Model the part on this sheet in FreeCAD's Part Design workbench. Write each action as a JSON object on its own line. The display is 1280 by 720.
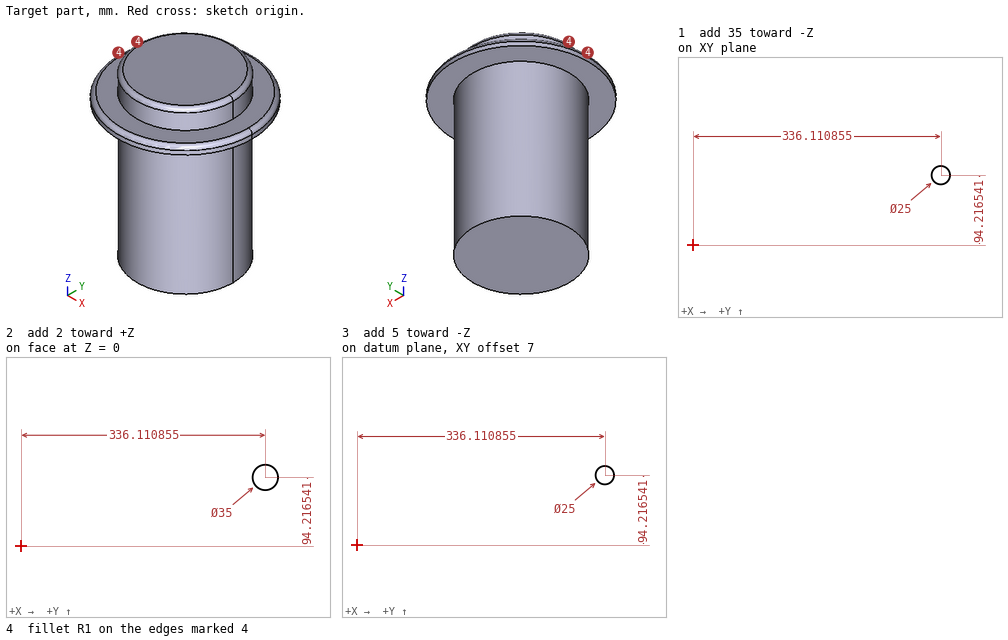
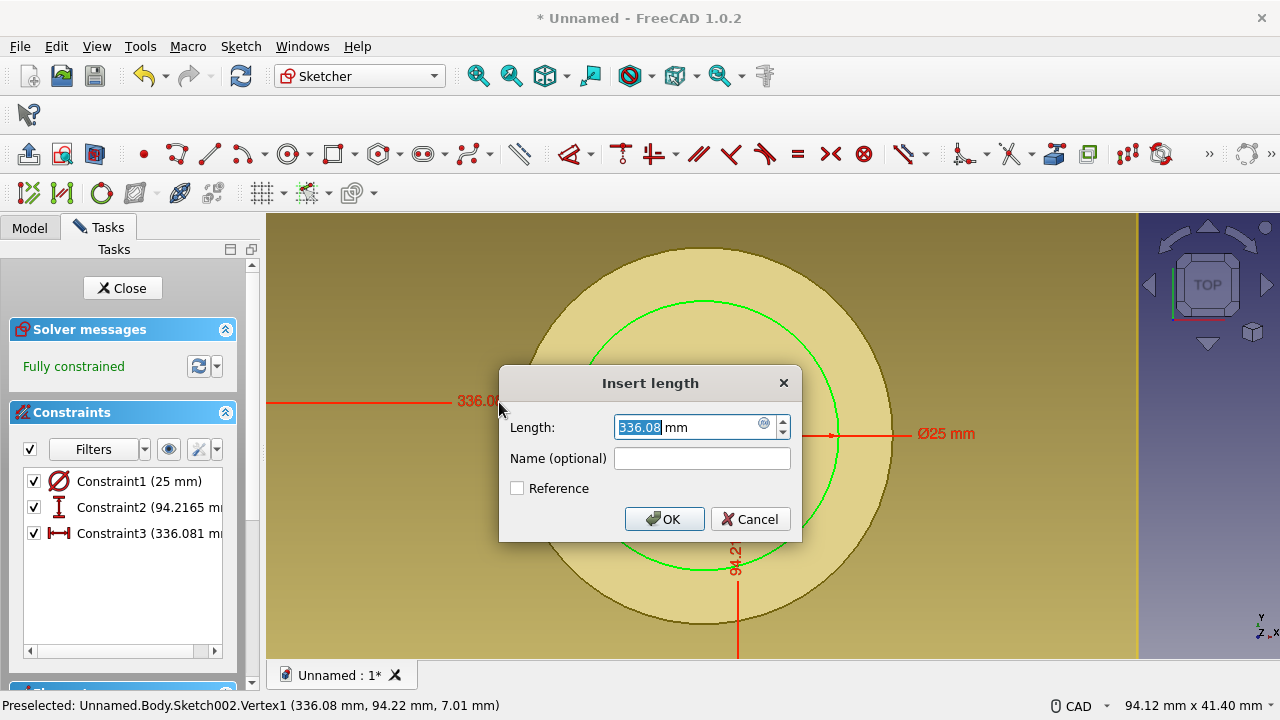
{"action": "type", "text": "336.110855"}
{"action": "key", "text": "Return"}
{"action": "key", "text": "Escape"}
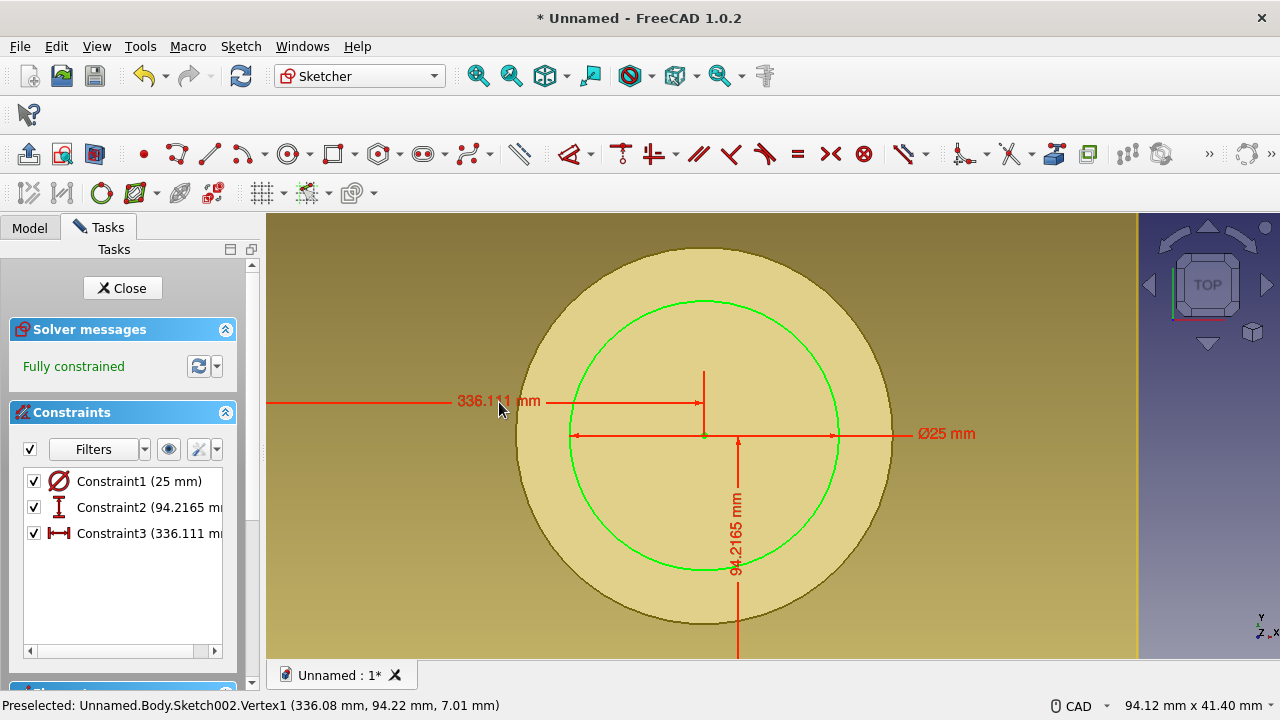
{"action": "left_click", "coordinate": [123, 288]}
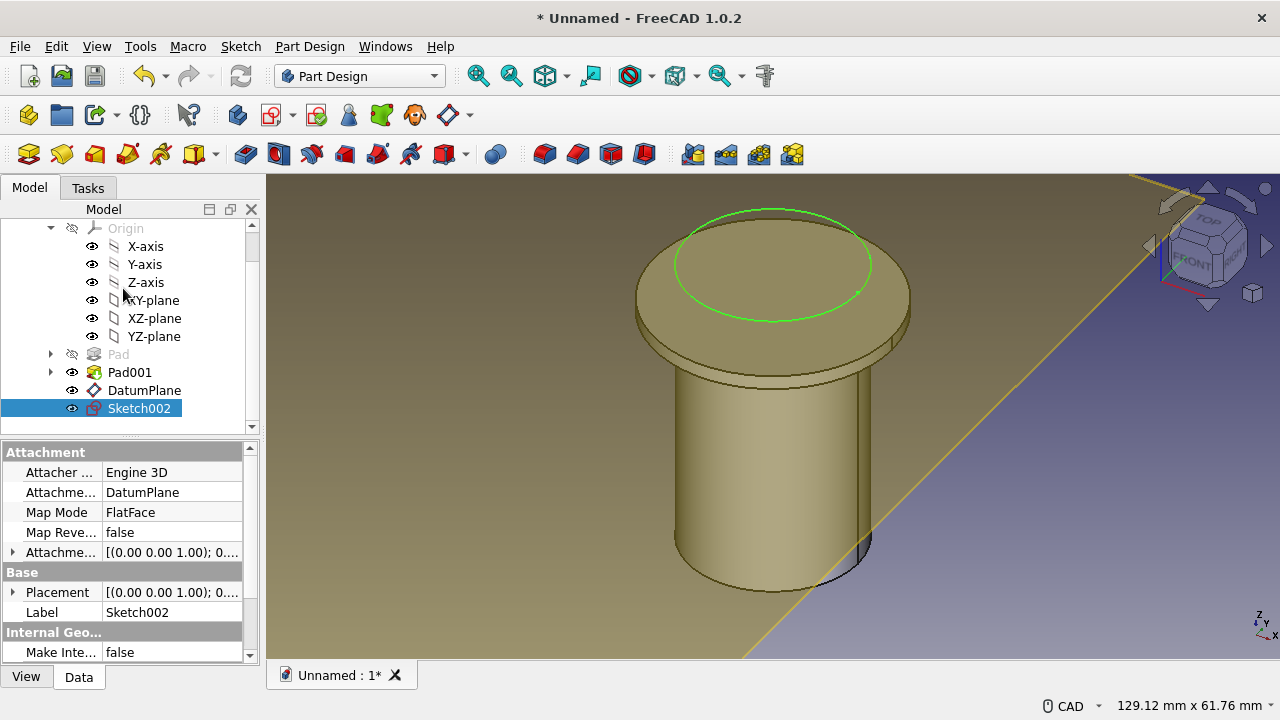
{"action": "left_click", "coordinate": [29, 154]}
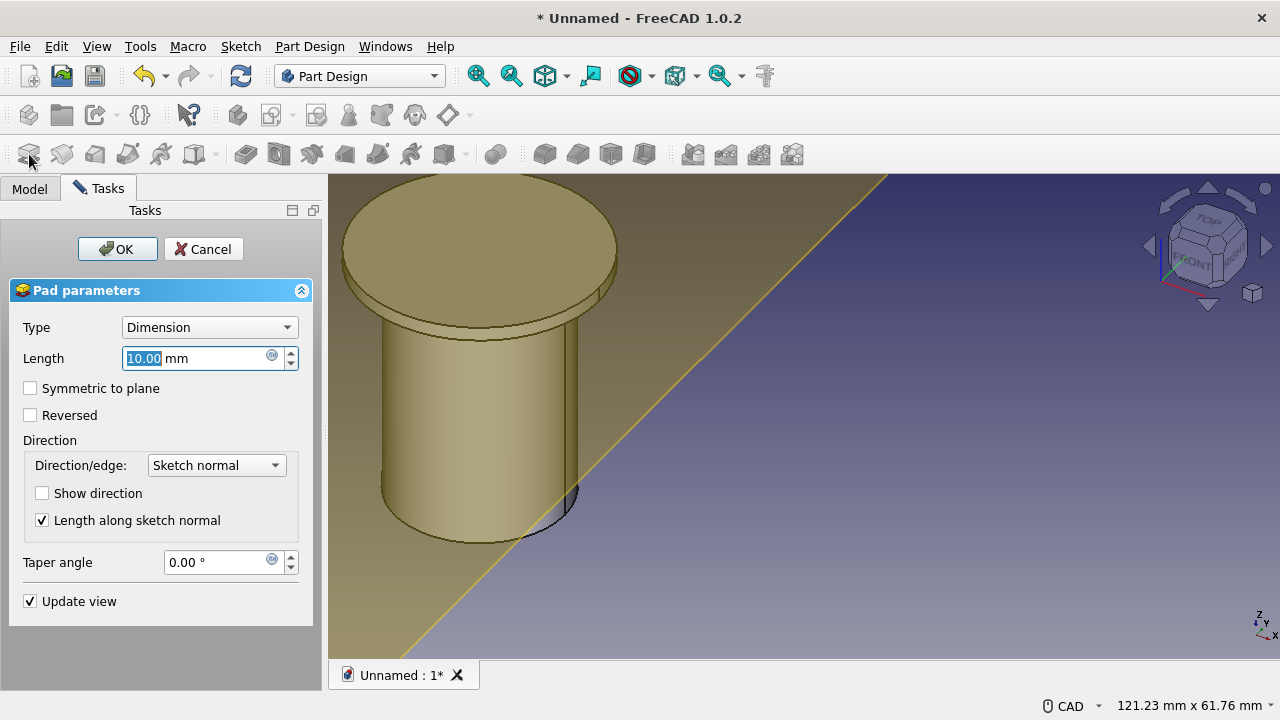
{"action": "type", "text": "5"}
{"action": "key", "text": "Tab"}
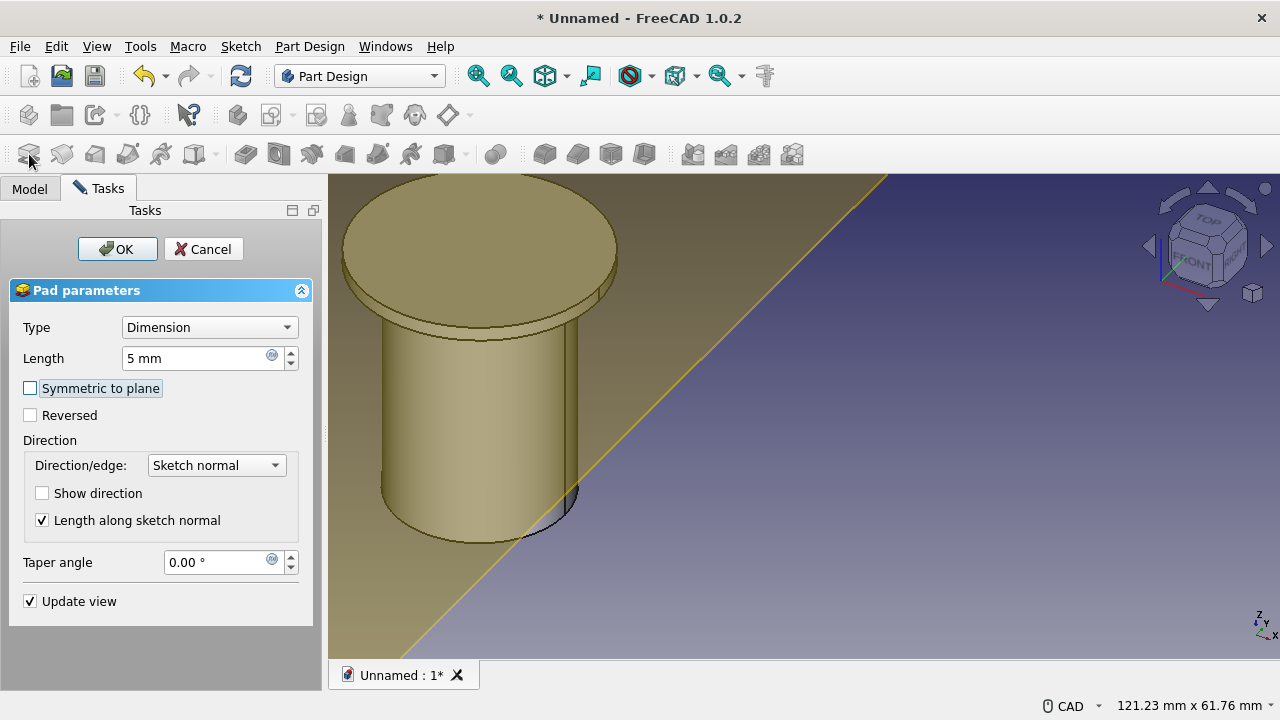
{"action": "left_click", "coordinate": [31, 415]}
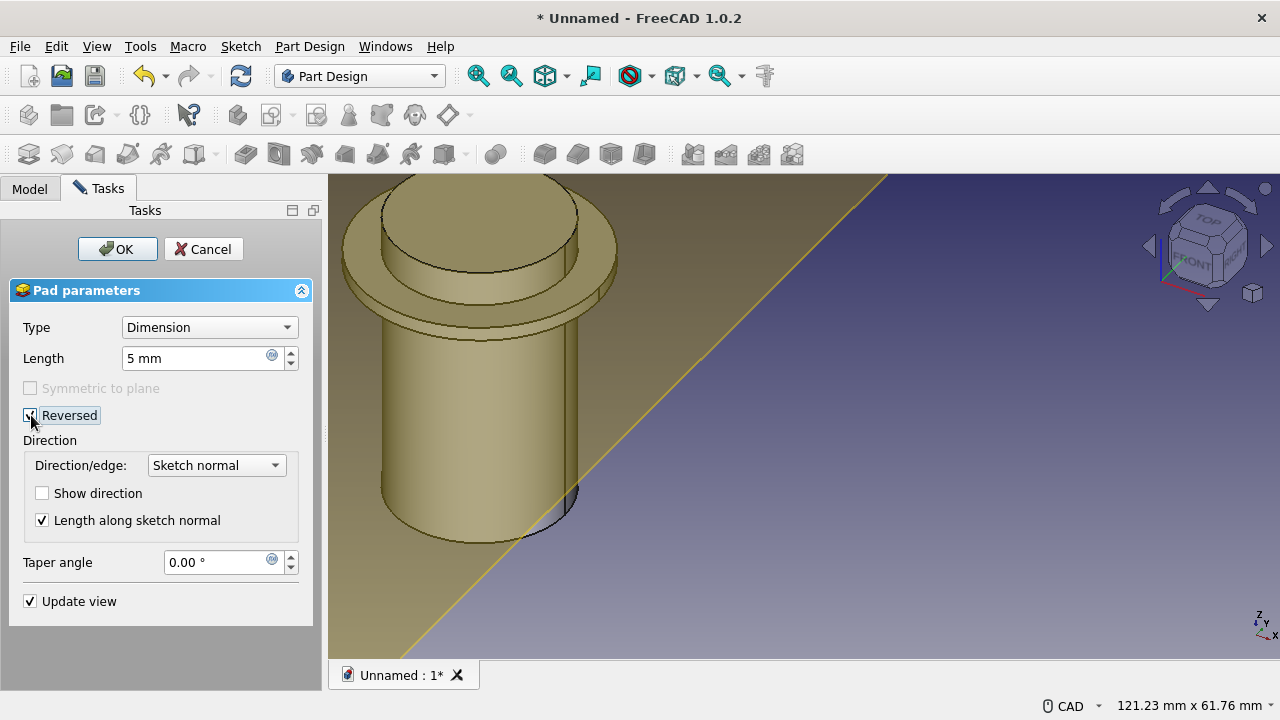
{"action": "left_click", "coordinate": [118, 249]}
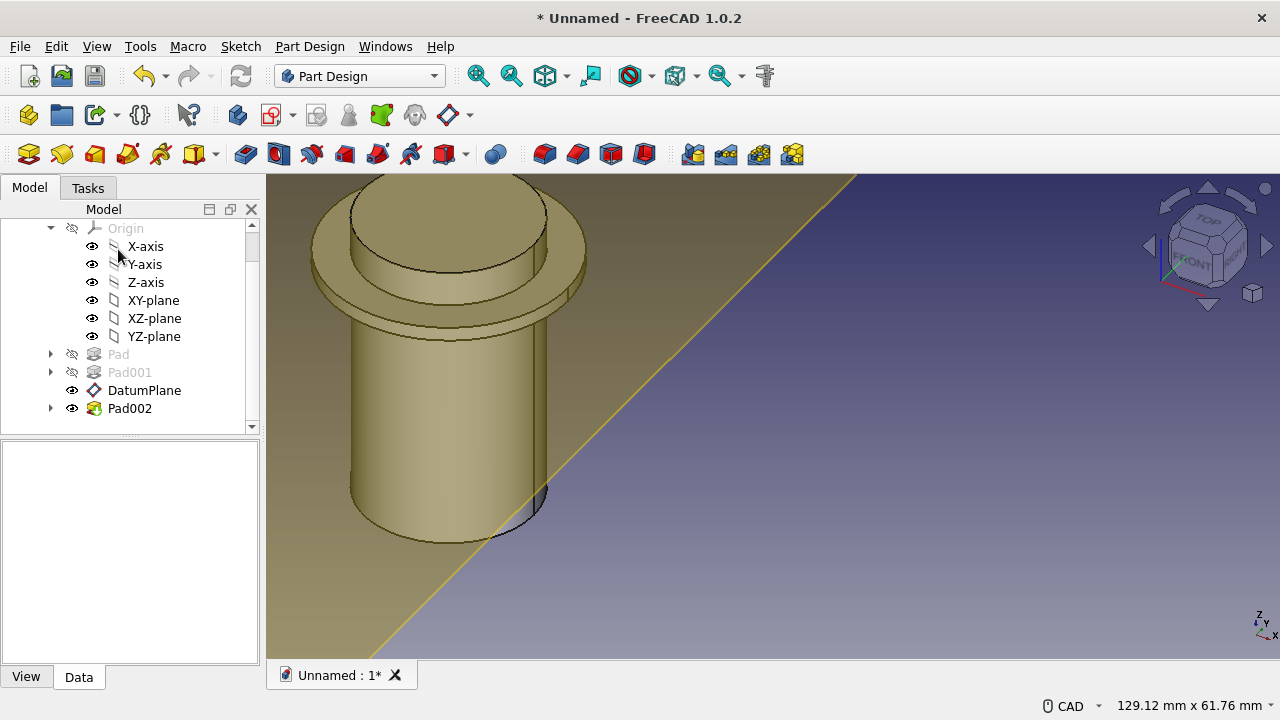
{"action": "left_click", "coordinate": [117, 390]}
{"action": "key", "text": "space"}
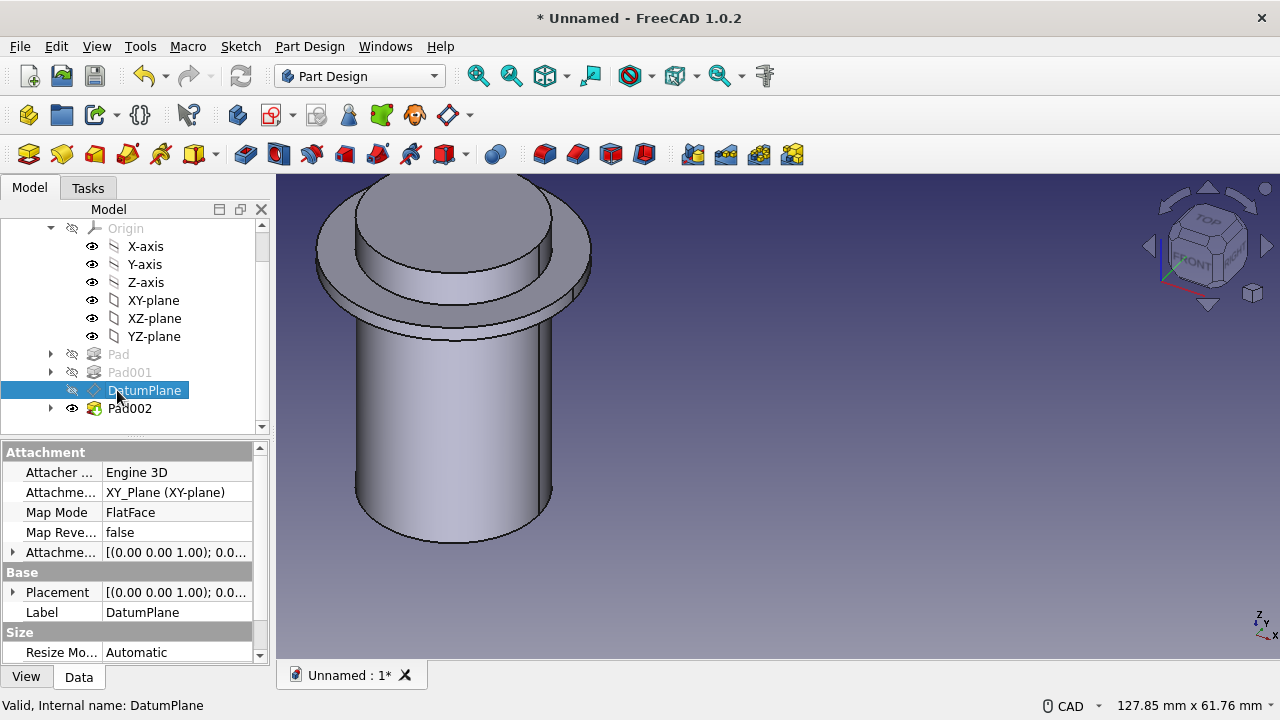
{"action": "left_click", "coordinate": [479, 76]}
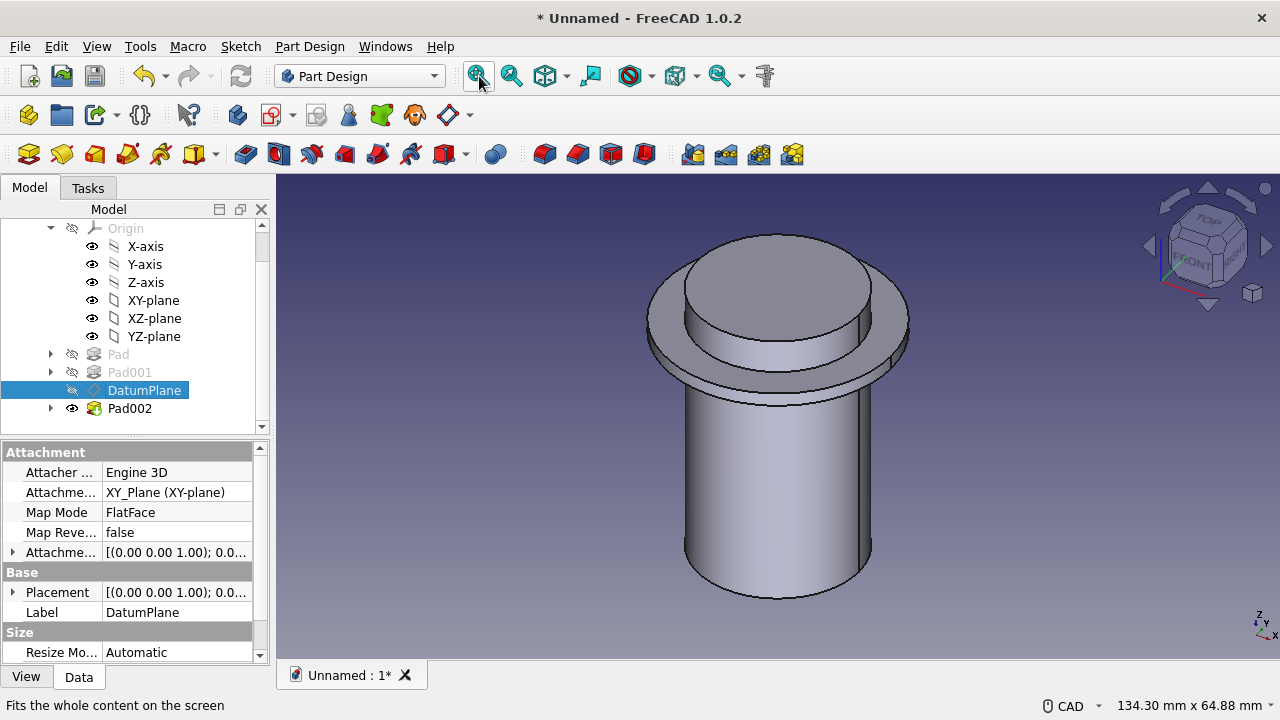
{"action": "left_click", "coordinate": [685, 293]}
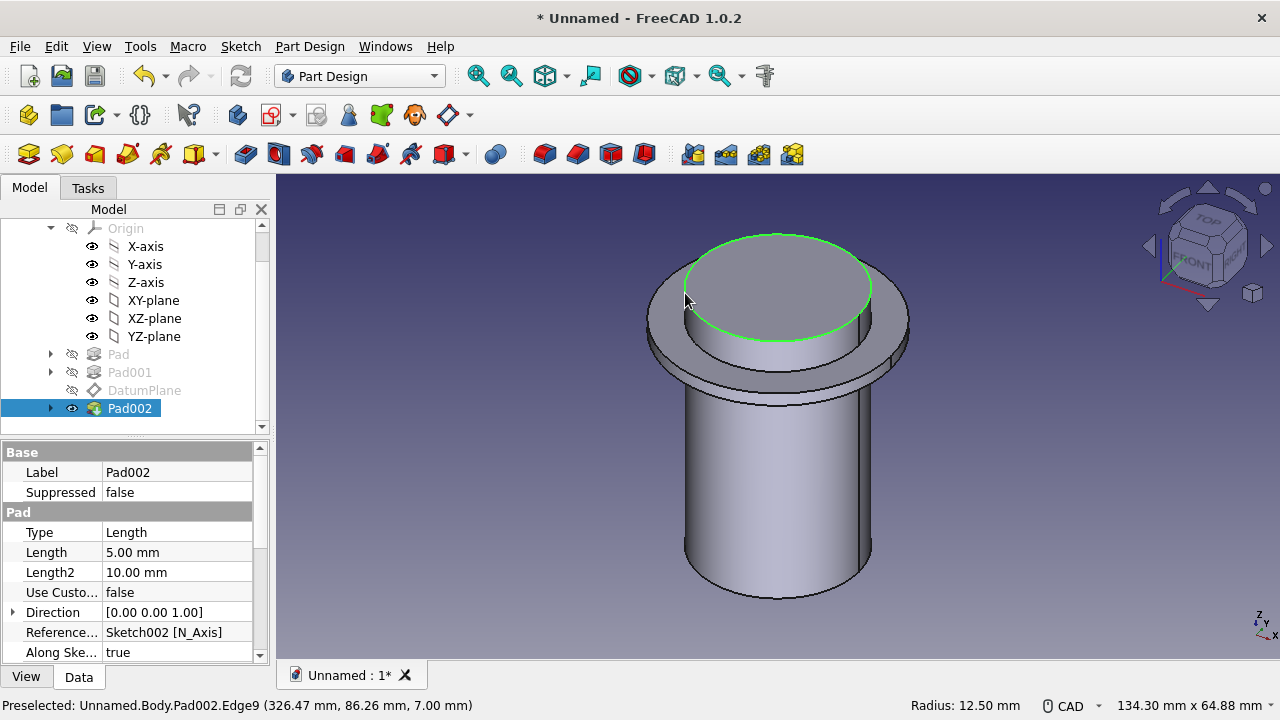
{"action": "left_click", "coordinate": [648, 325], "text": "ctrl"}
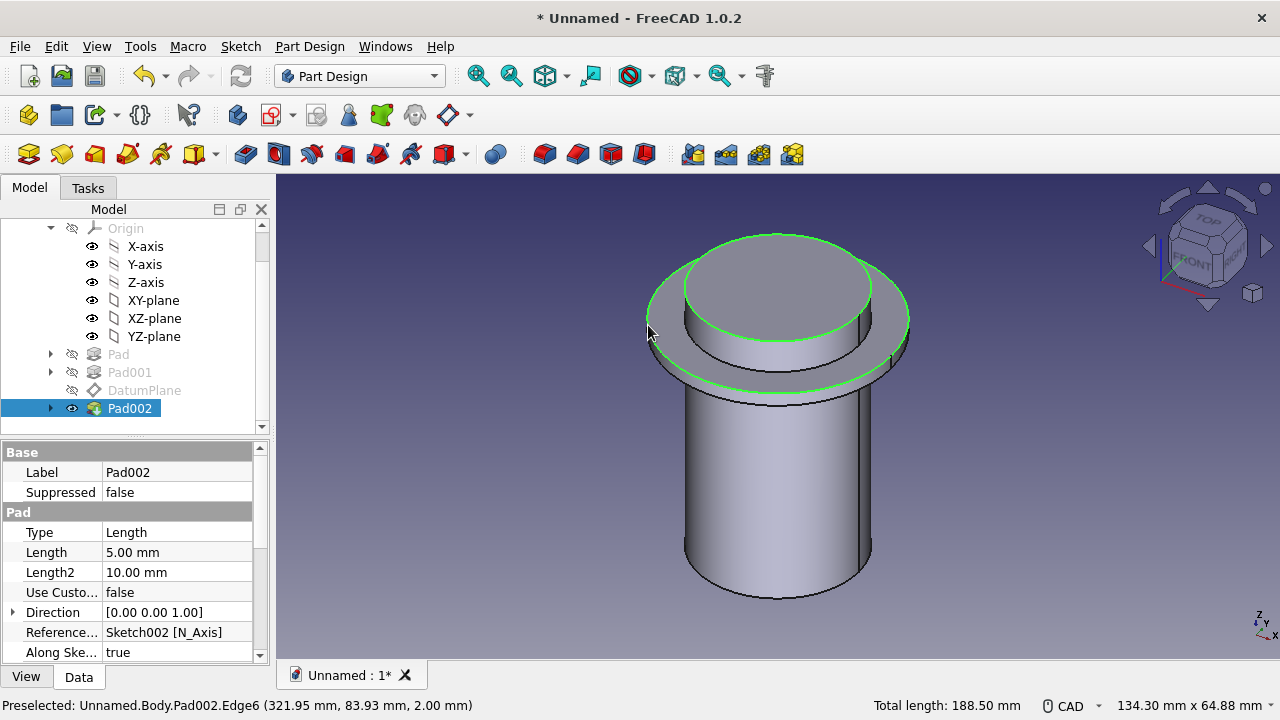
{"action": "left_click", "coordinate": [545, 154]}